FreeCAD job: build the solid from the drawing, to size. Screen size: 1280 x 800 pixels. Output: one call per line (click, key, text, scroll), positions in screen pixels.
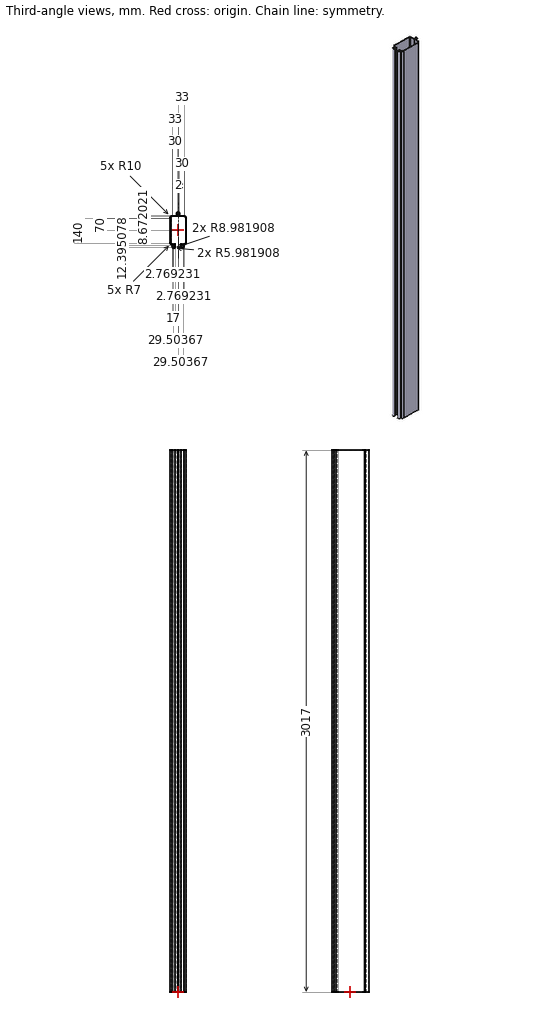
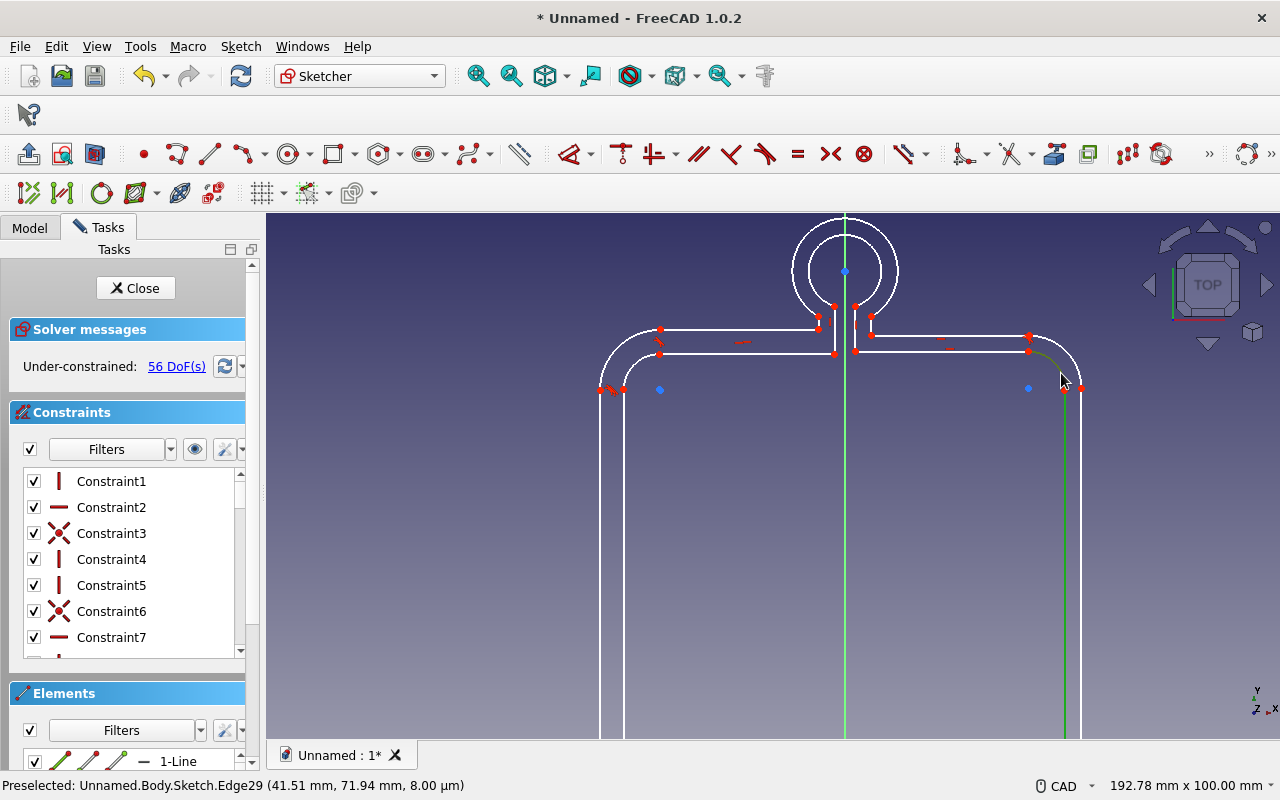
click(765, 154)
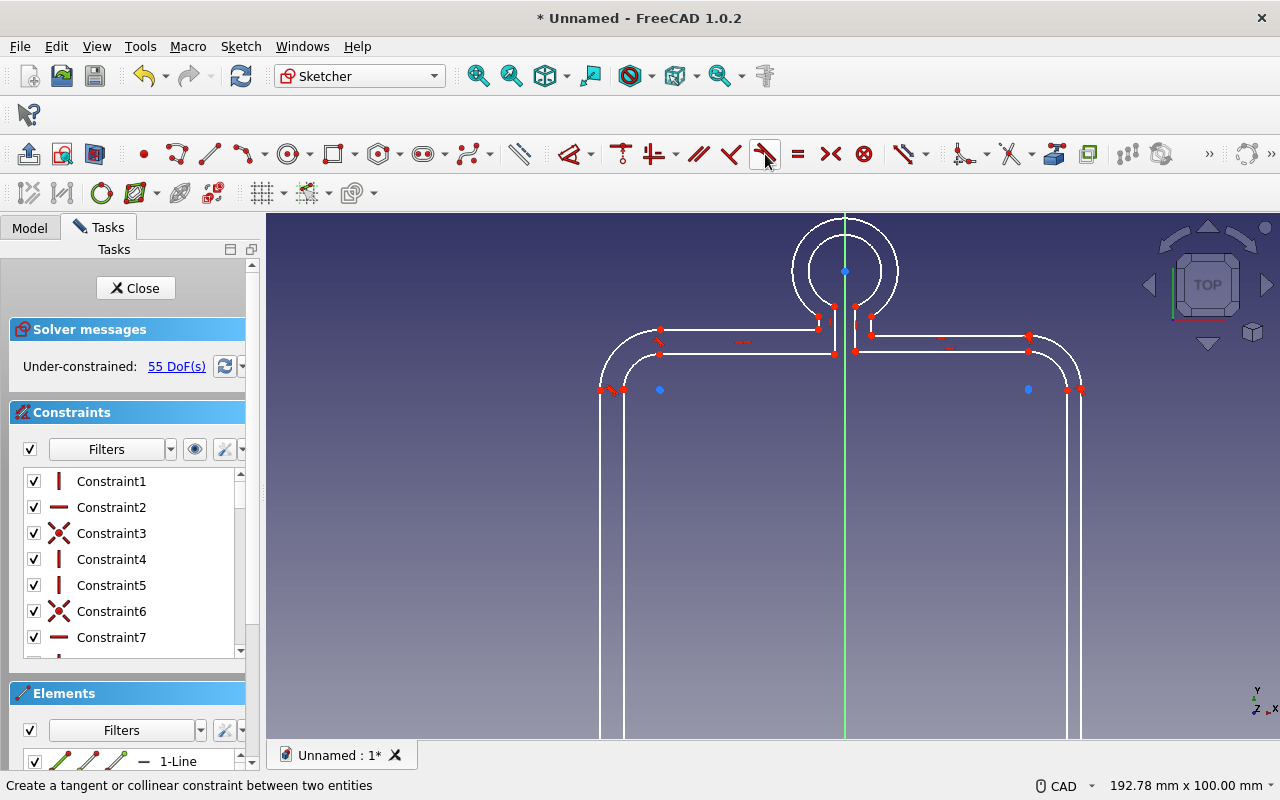
click(1067, 612)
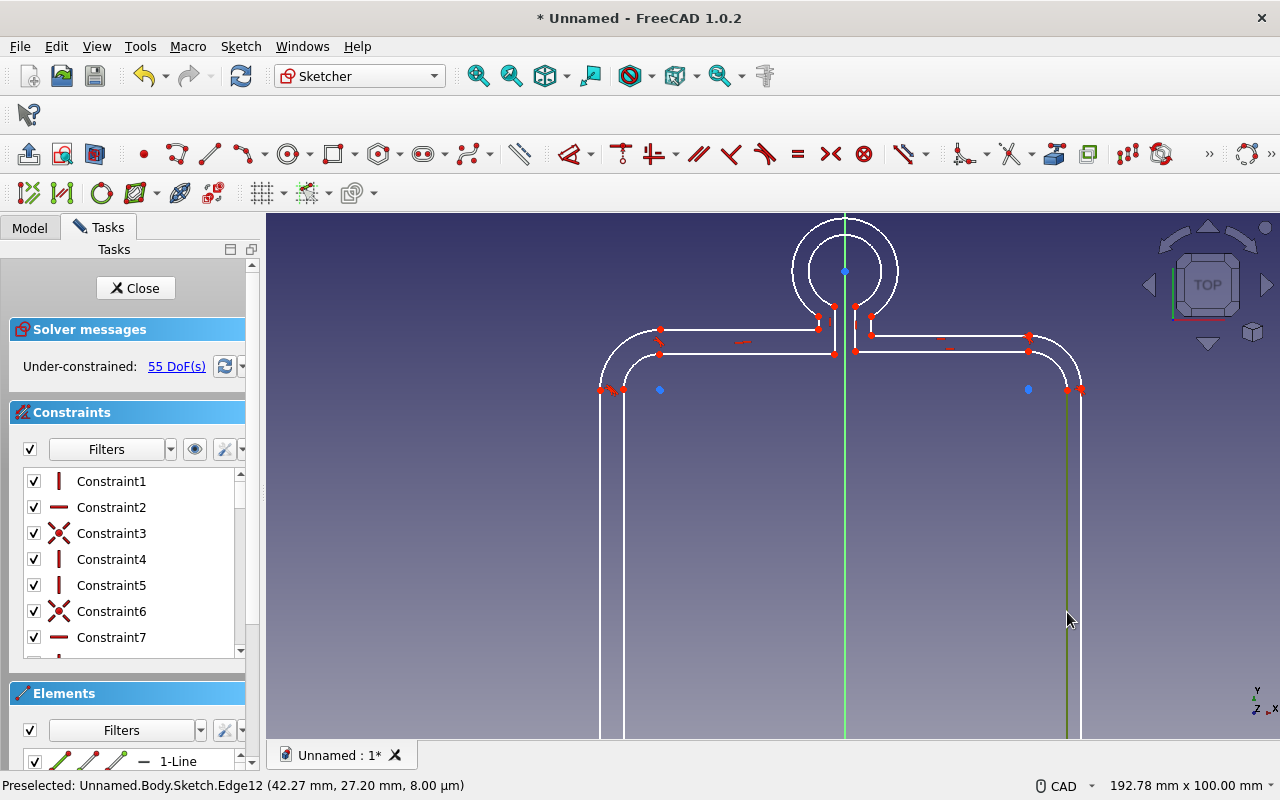
scroll(644, 357, down, 6)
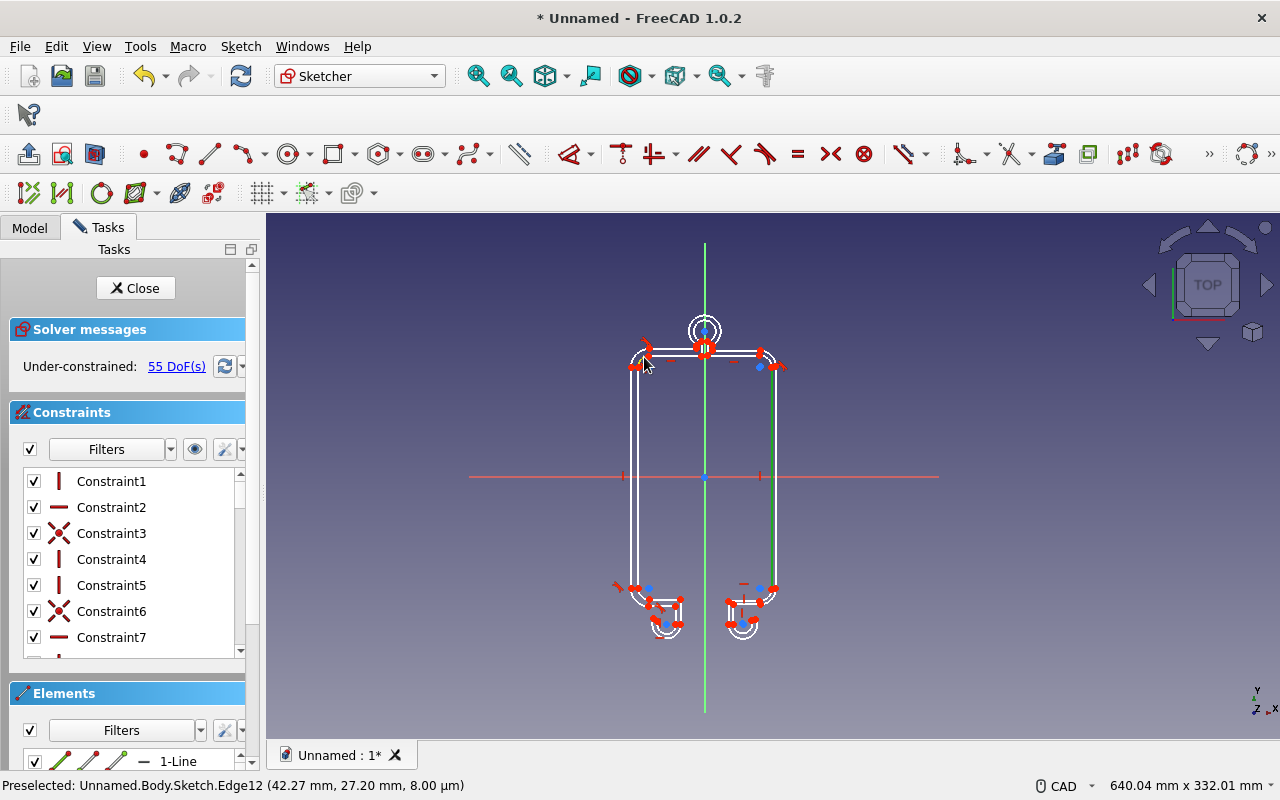
scroll(765, 600, up, 7)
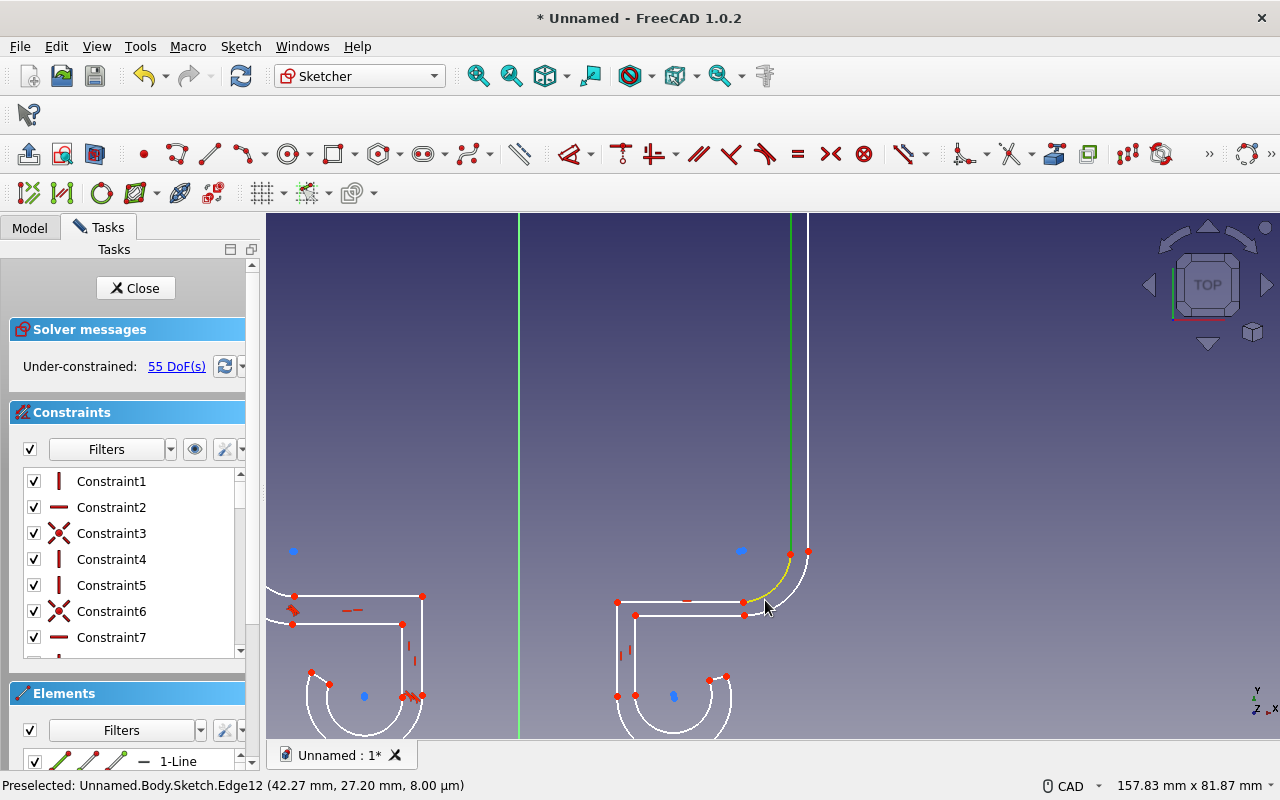
click(764, 596)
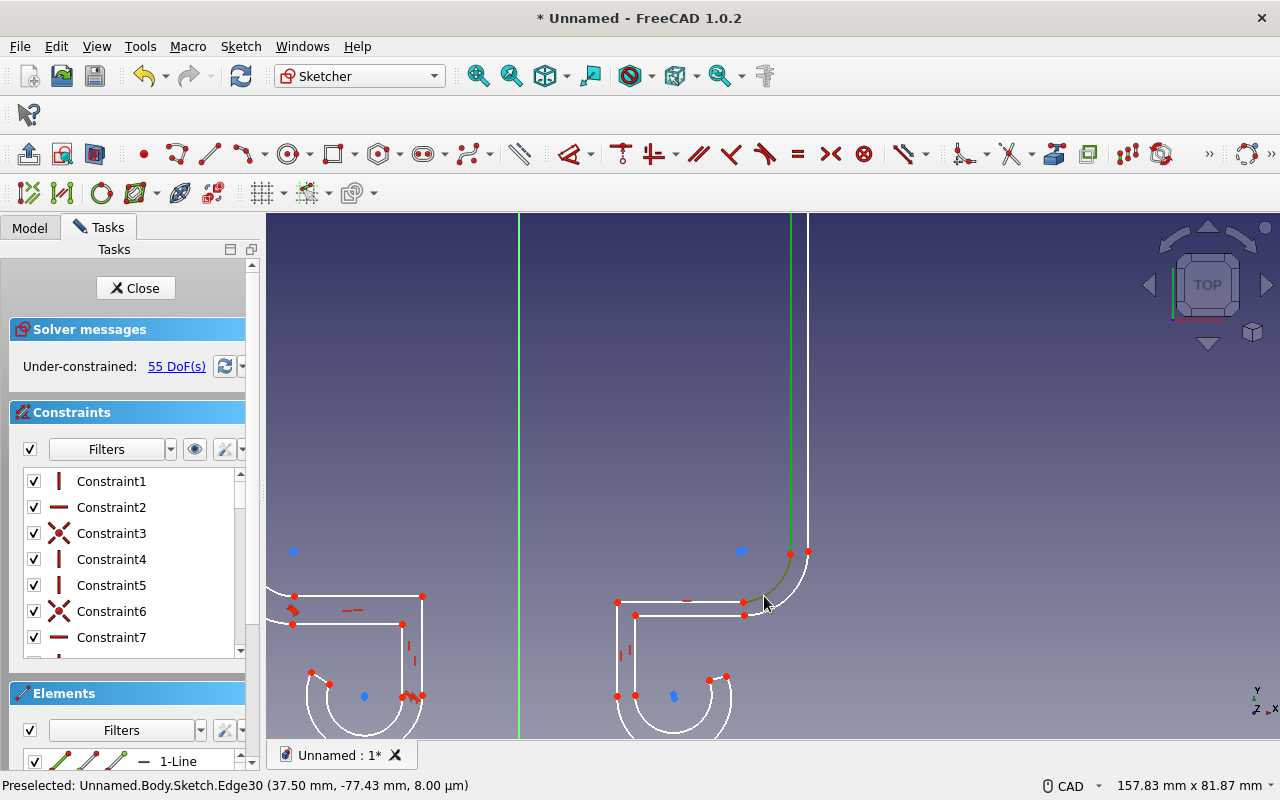
click(765, 154)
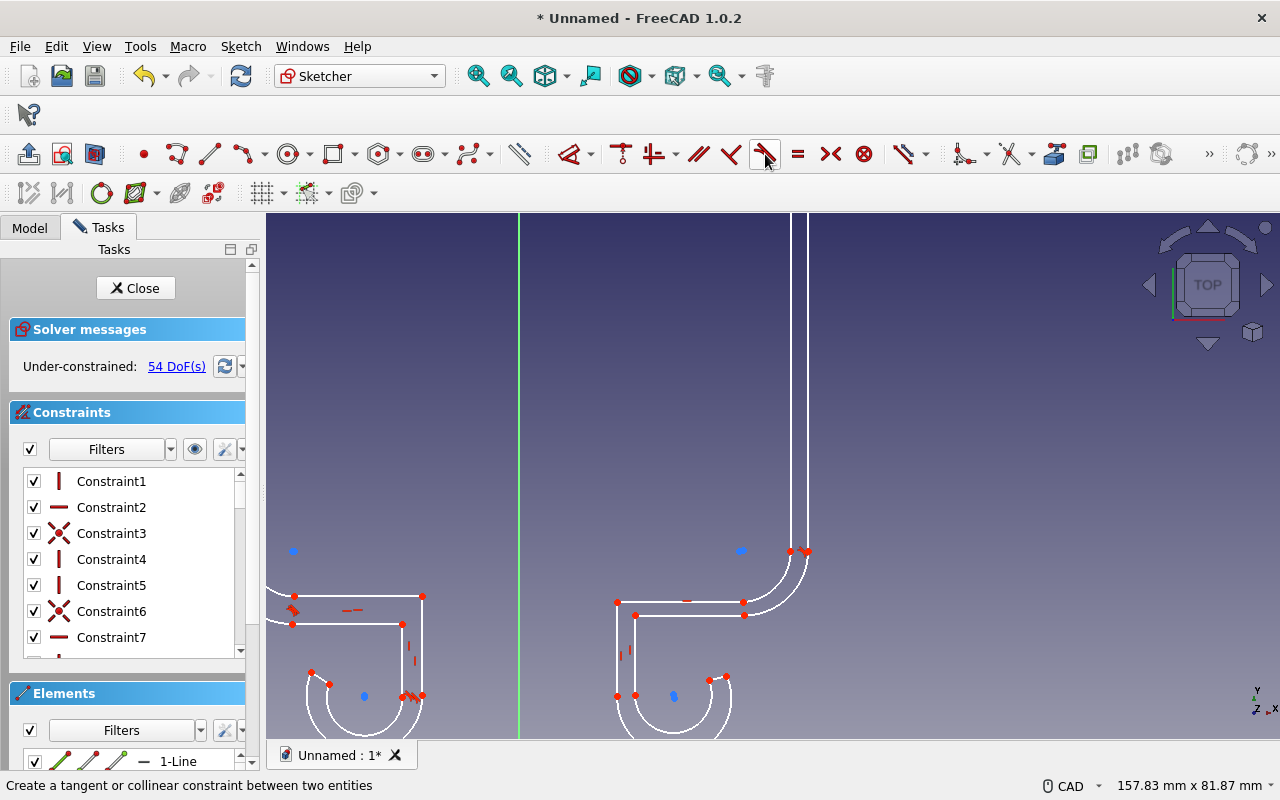
click(705, 602)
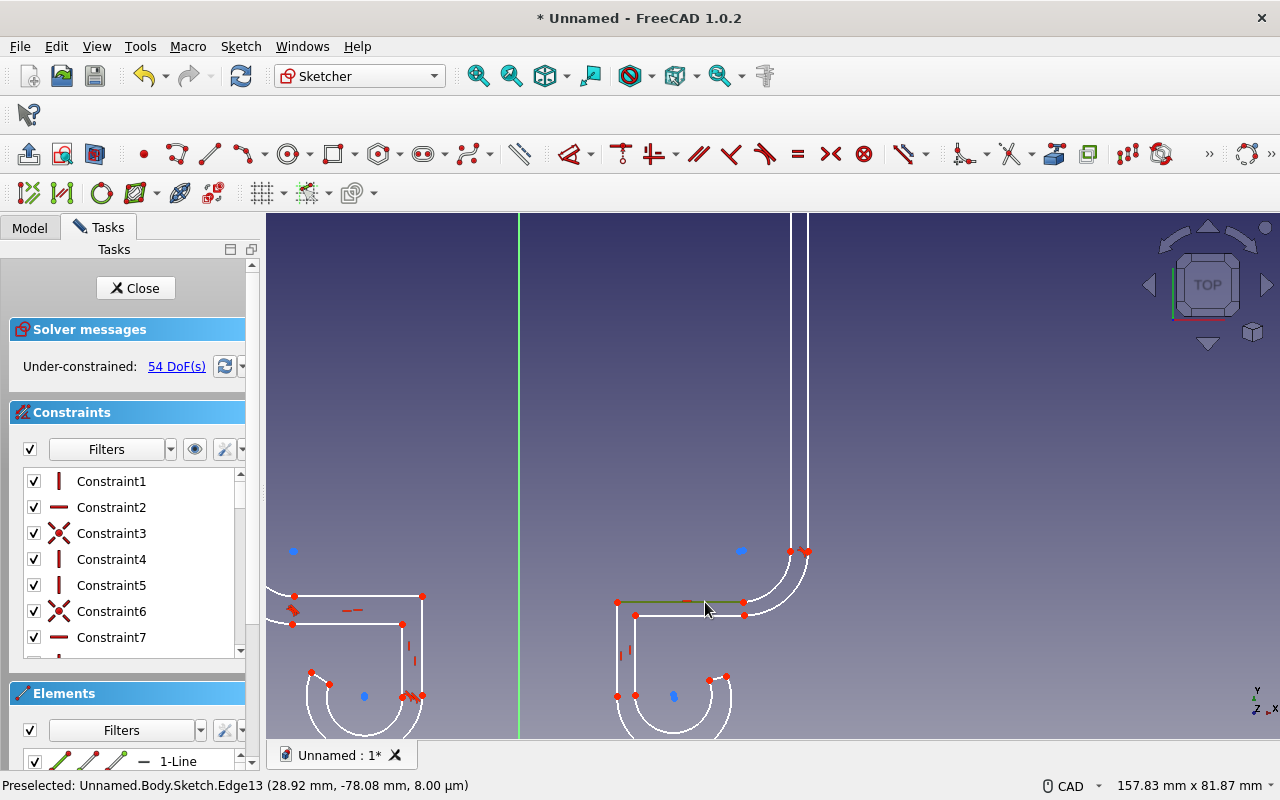
click(765, 596)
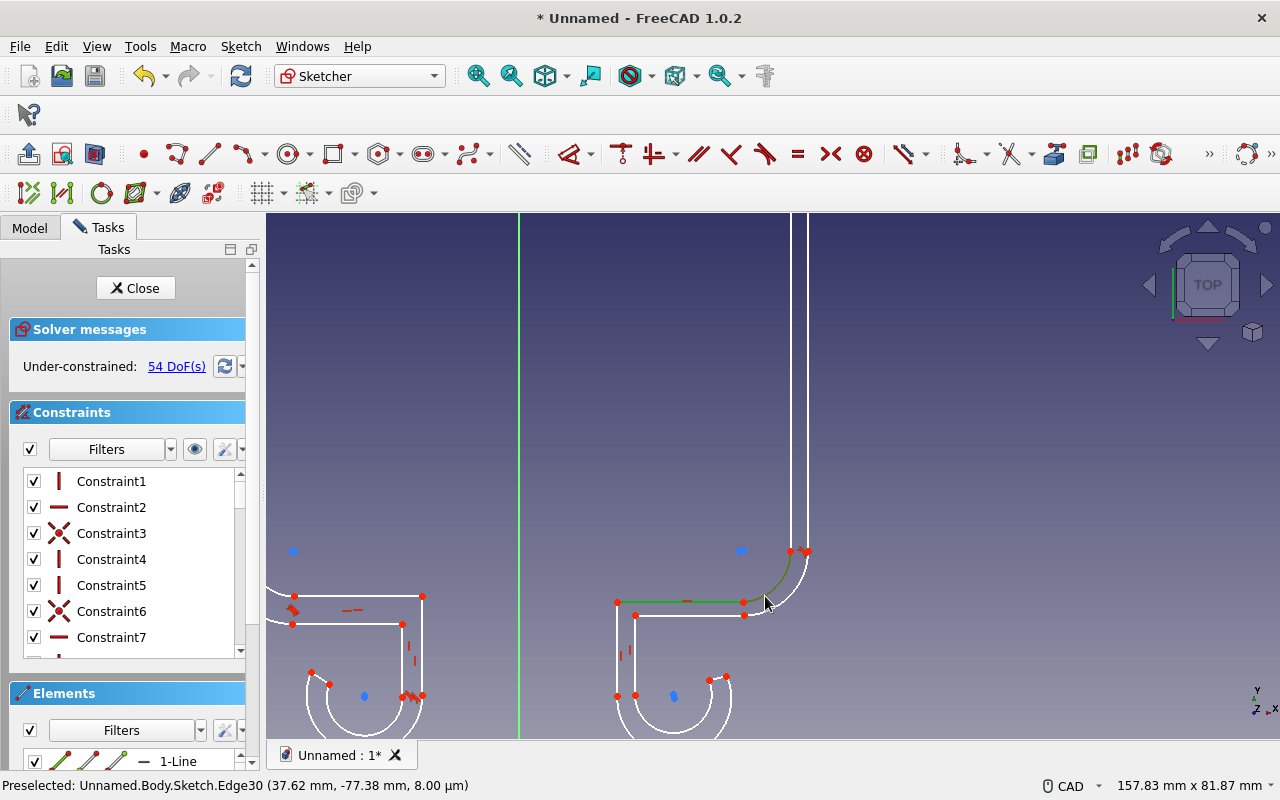
click(765, 154)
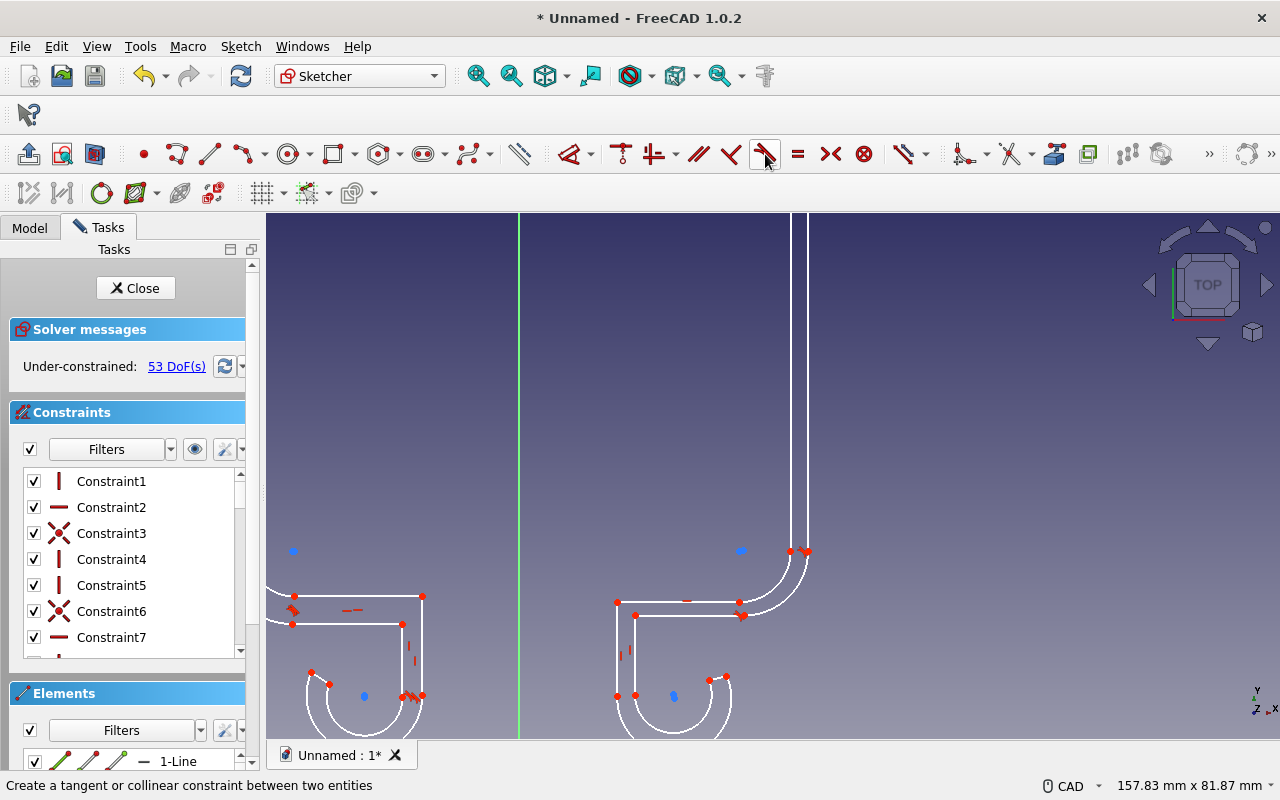
click(617, 630)